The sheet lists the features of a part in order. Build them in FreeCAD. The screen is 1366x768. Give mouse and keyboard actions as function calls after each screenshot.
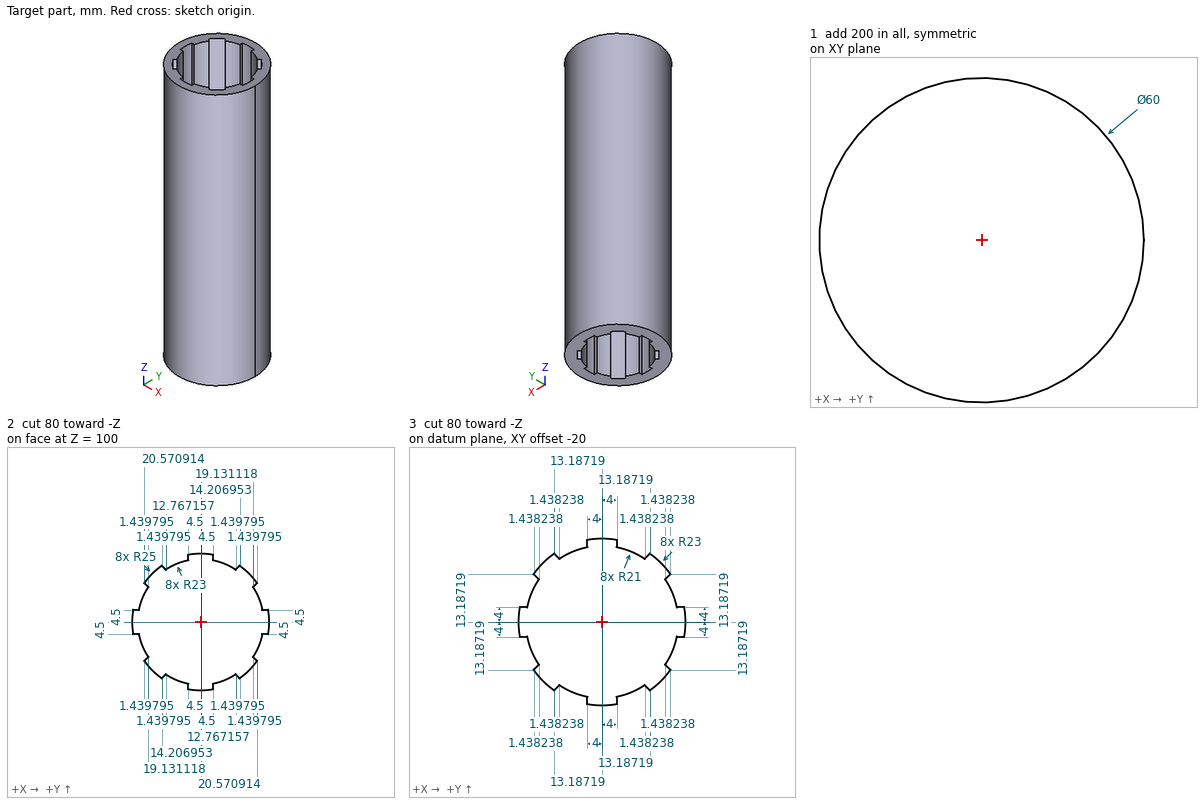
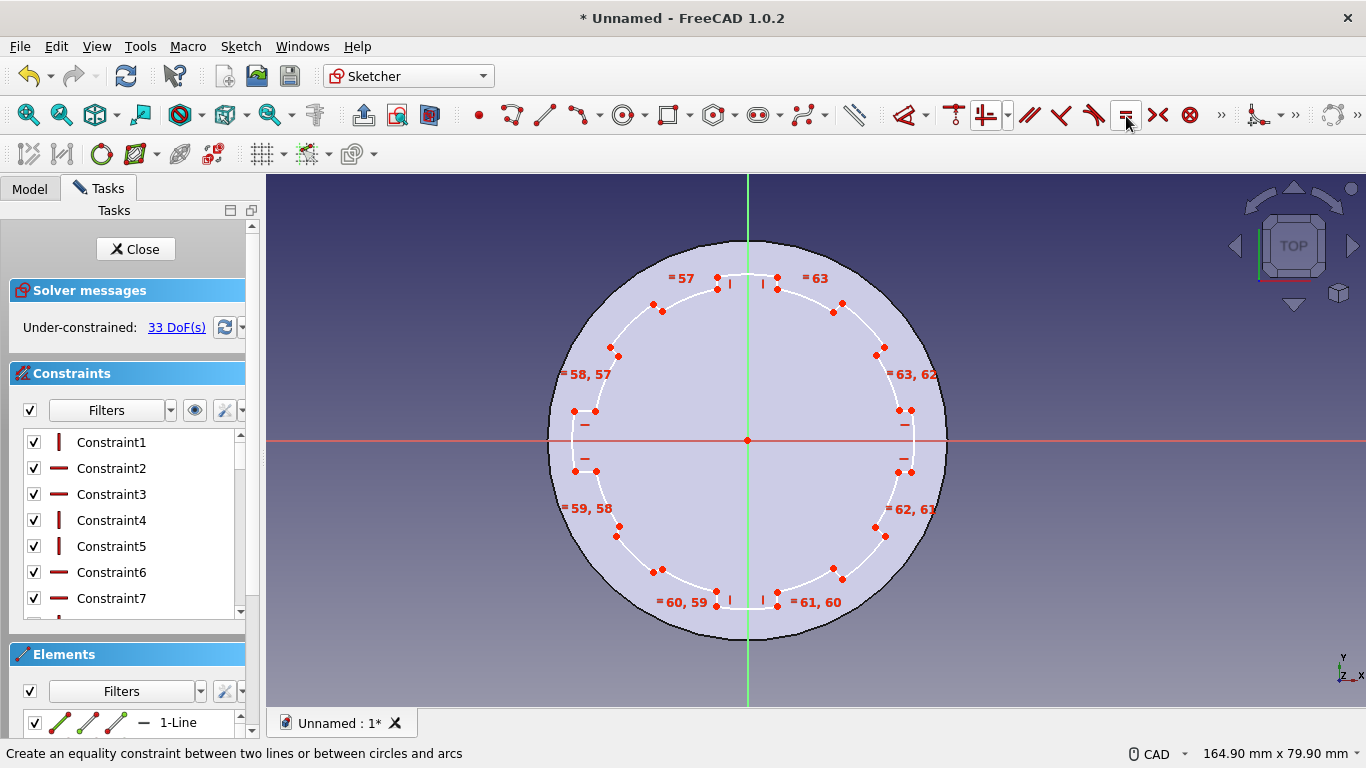
click(639, 315)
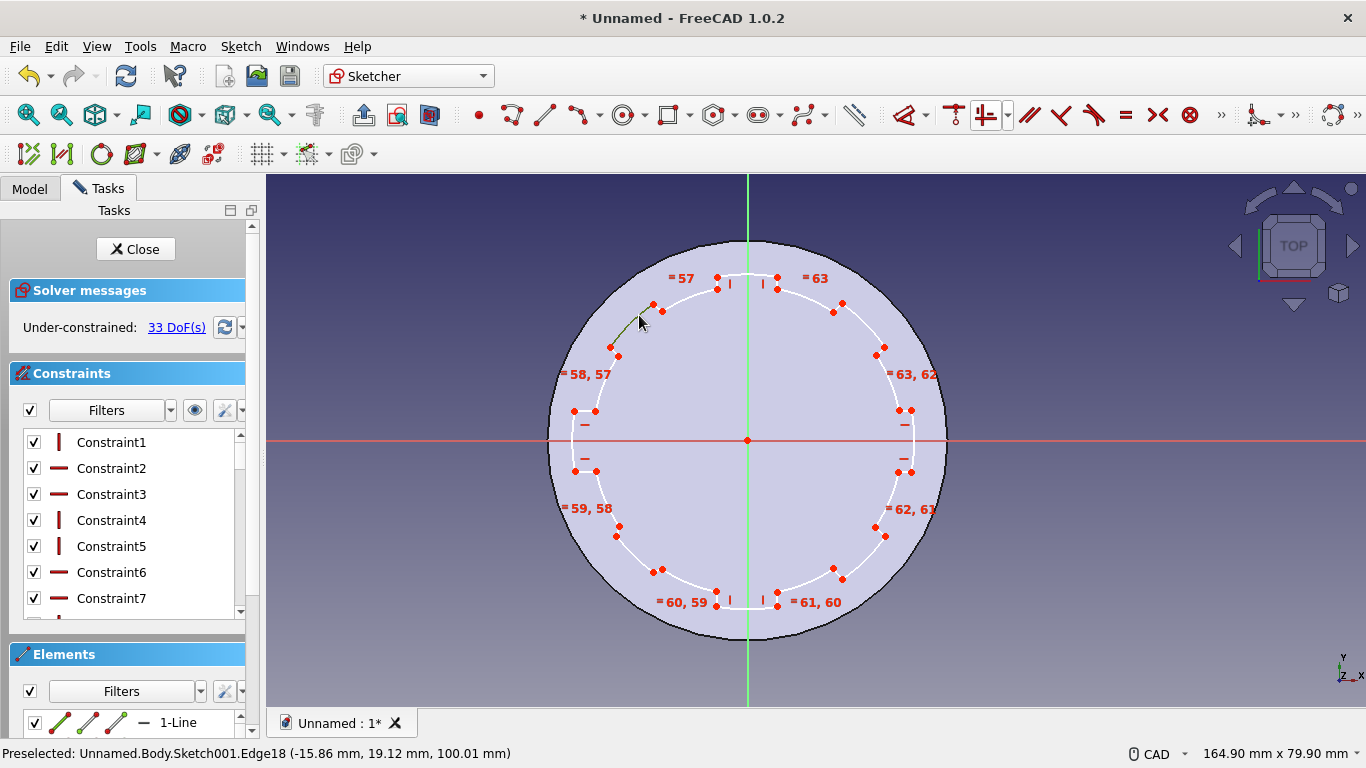
scroll(573, 429, up, 2)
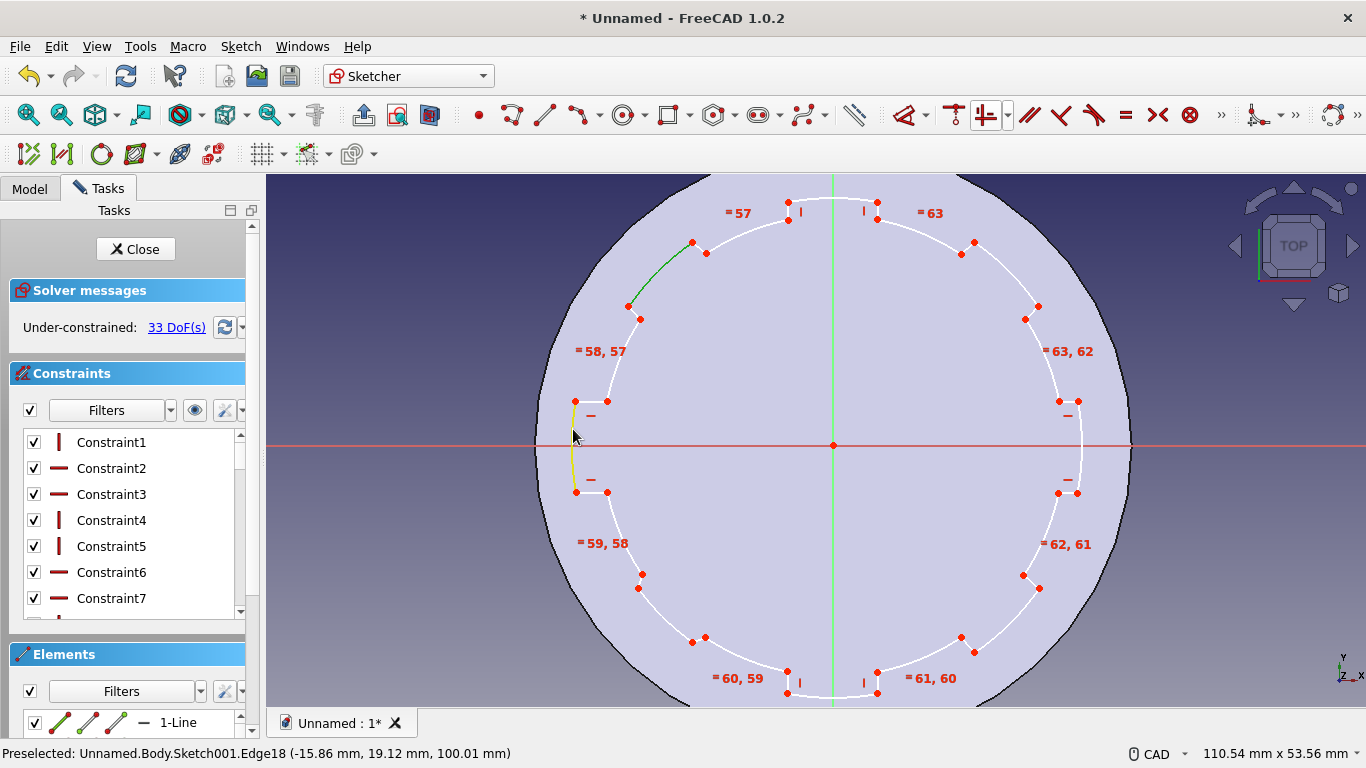
click(572, 429)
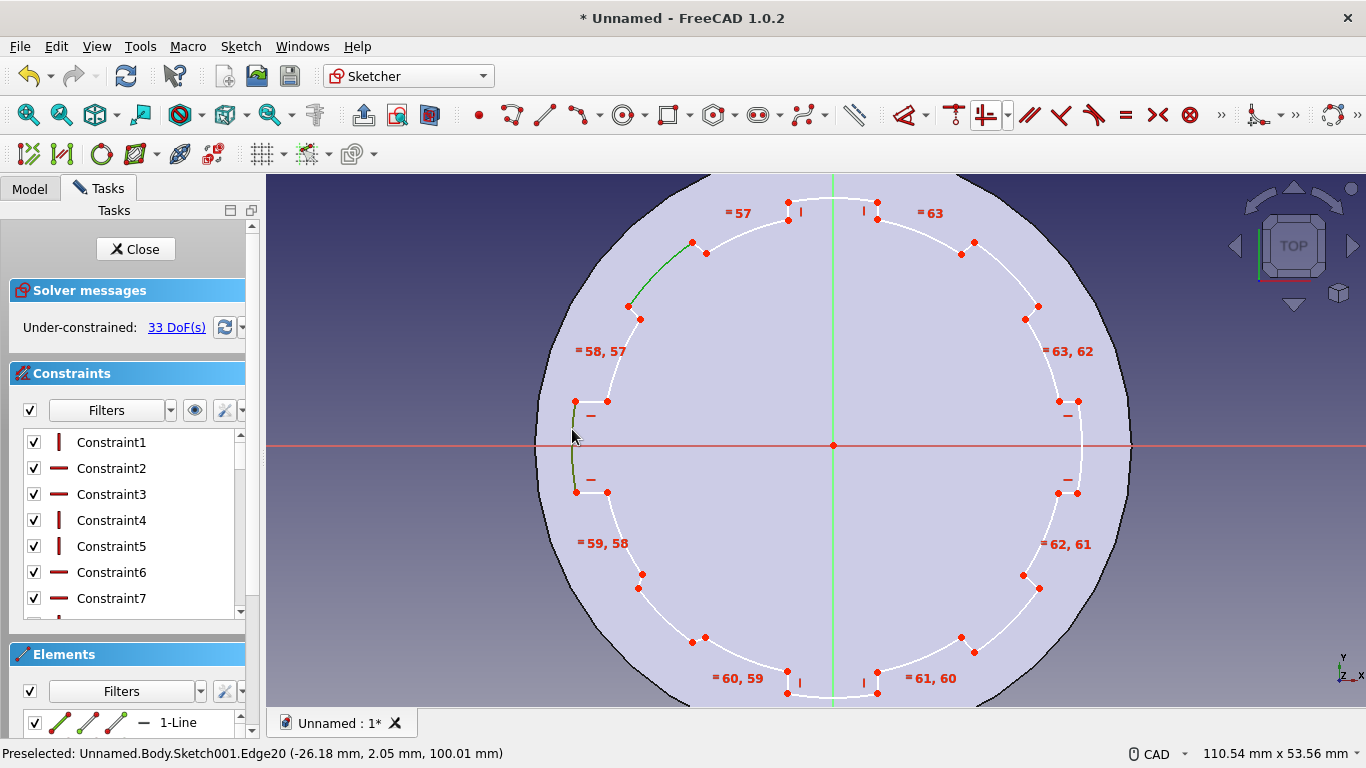
click(653, 606)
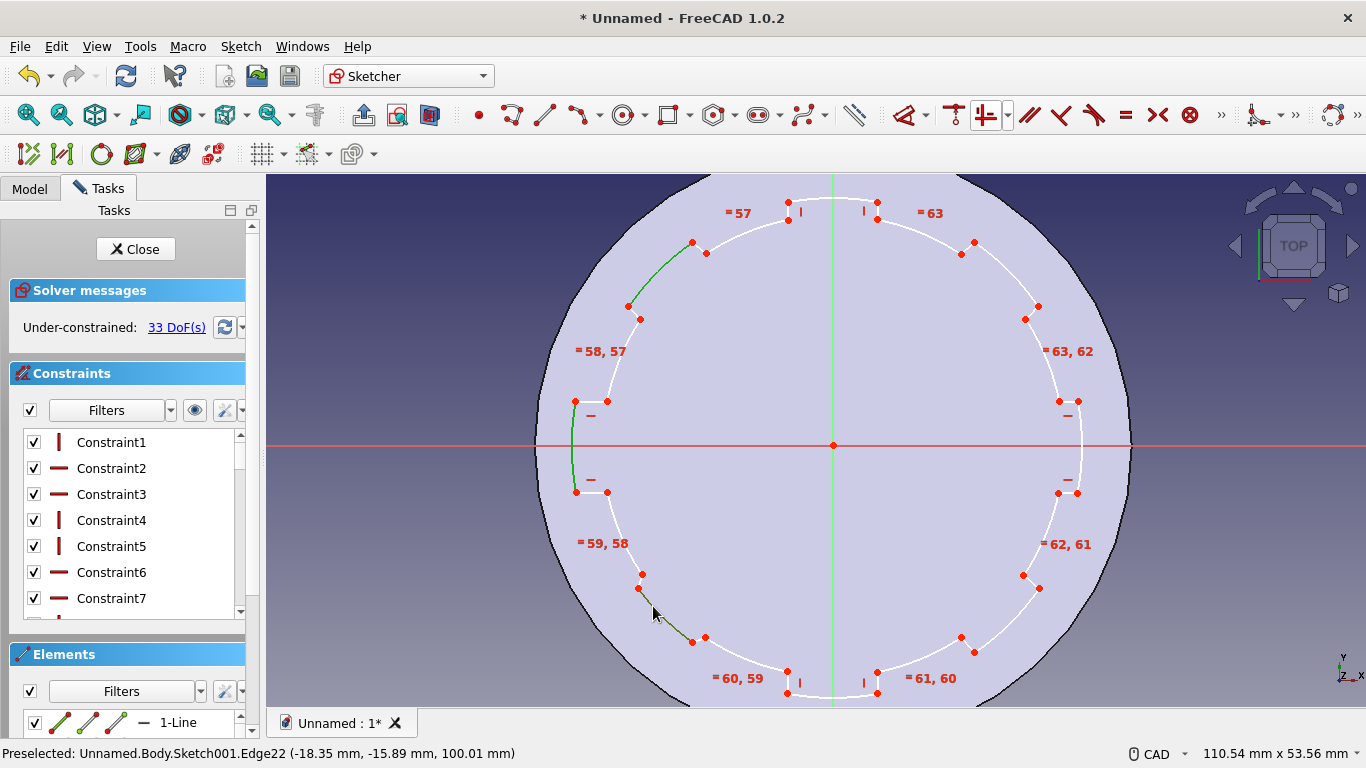
scroll(573, 429, down, 2)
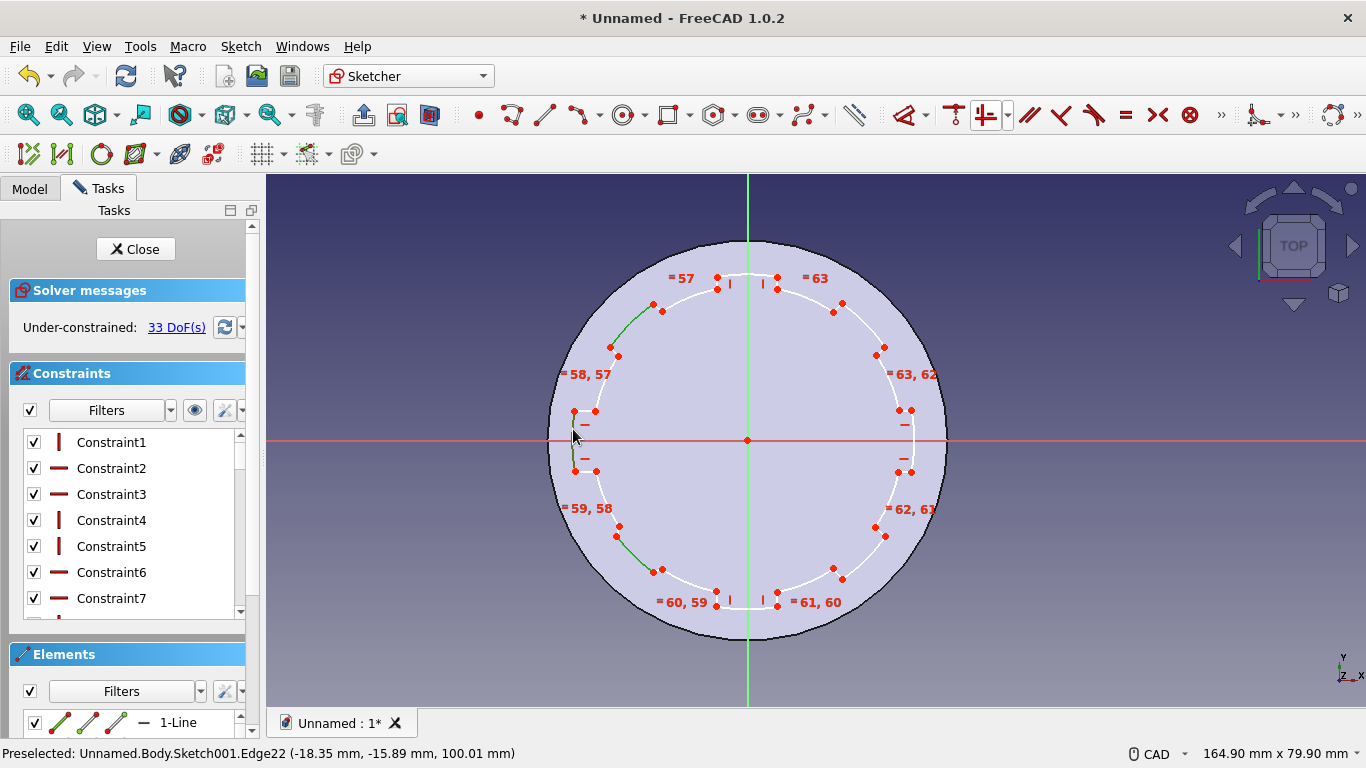
click(735, 609)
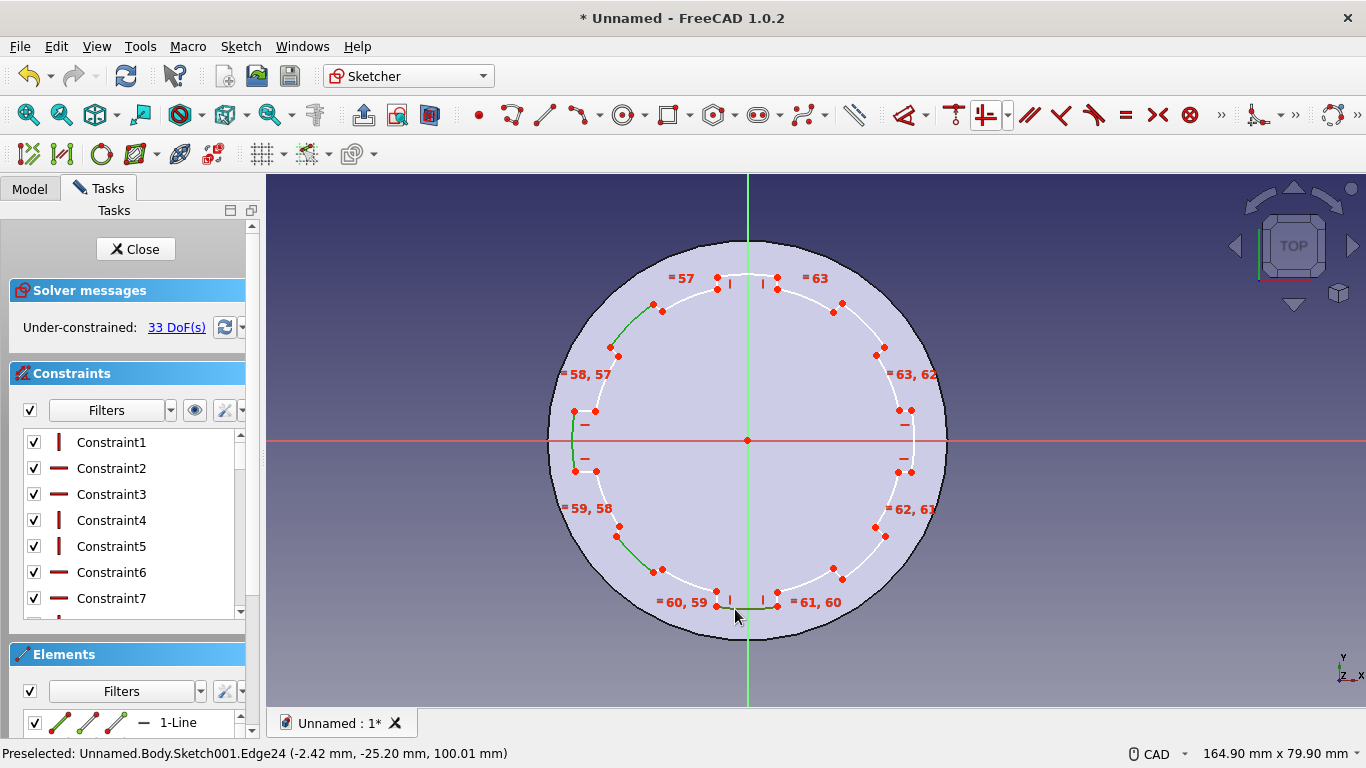
click(857, 568)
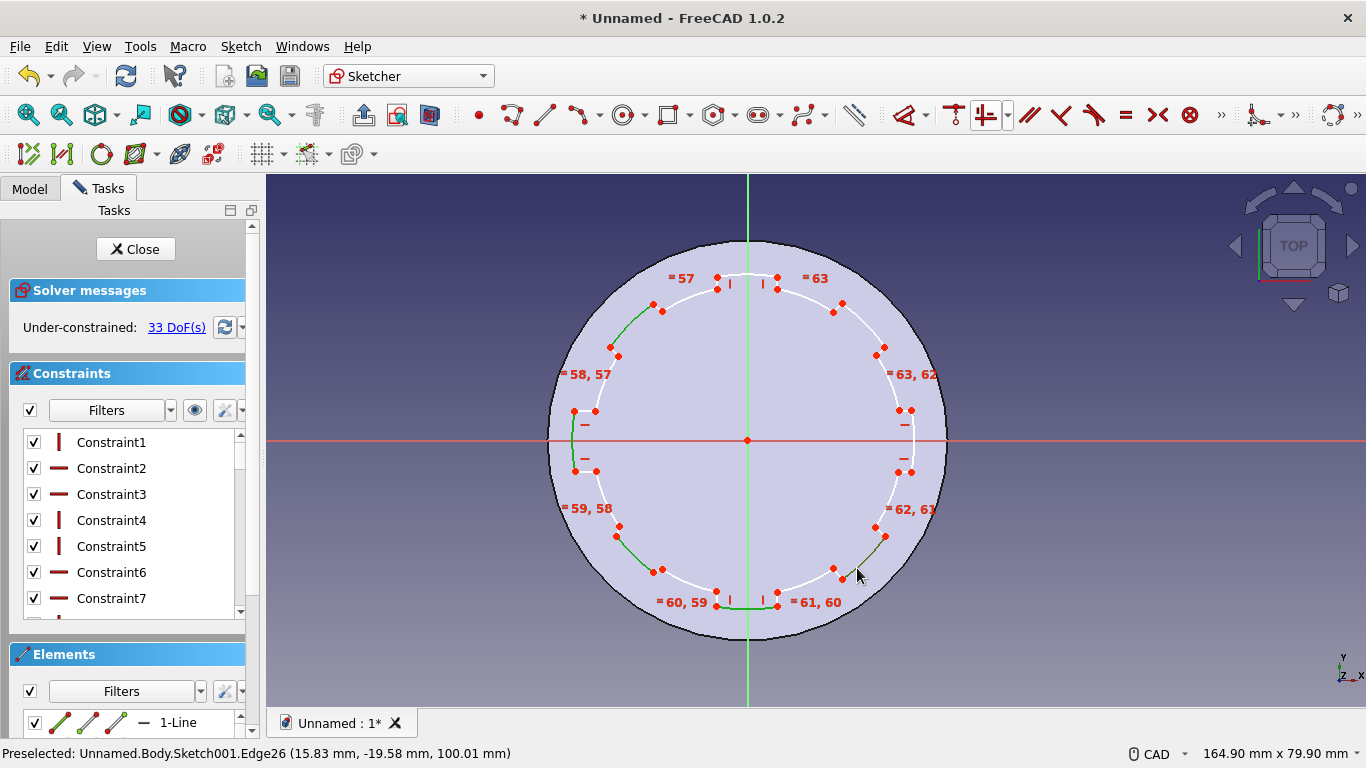
click(914, 454)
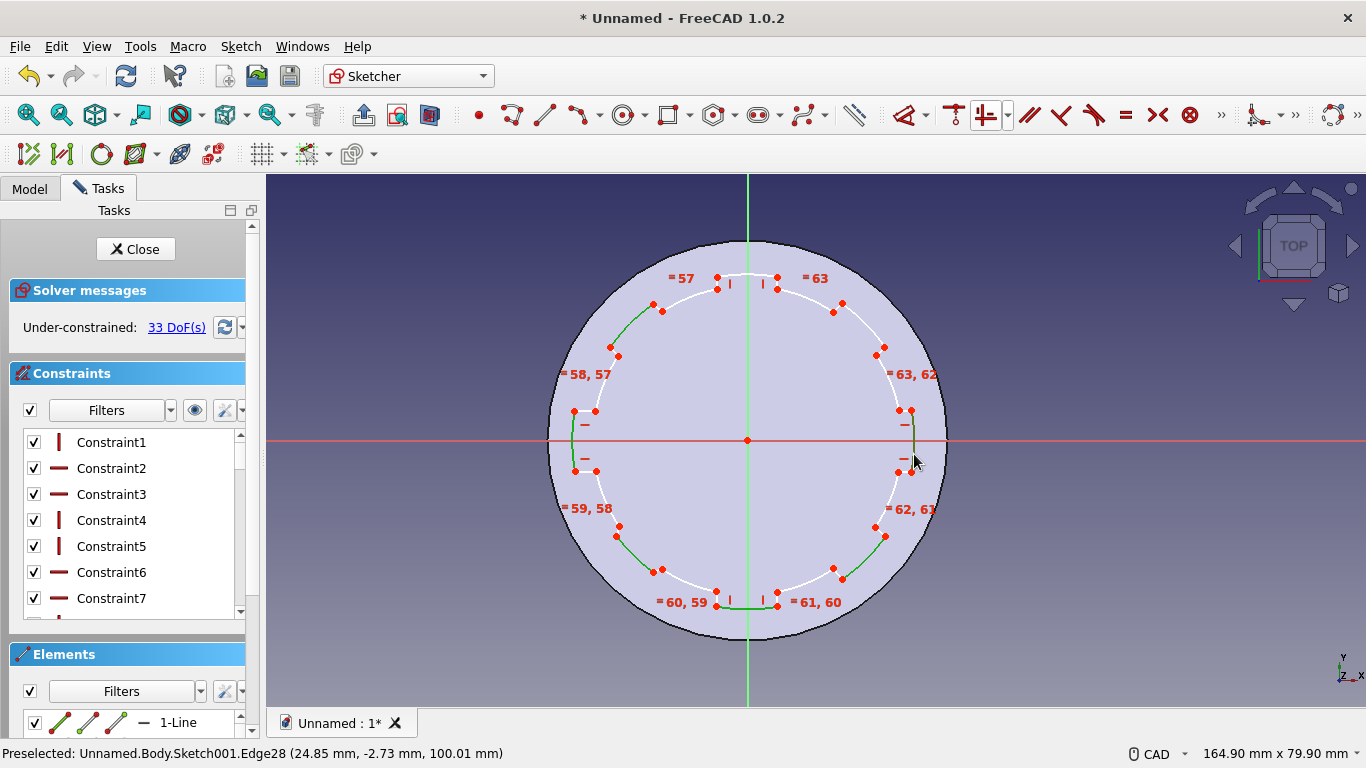
click(874, 333)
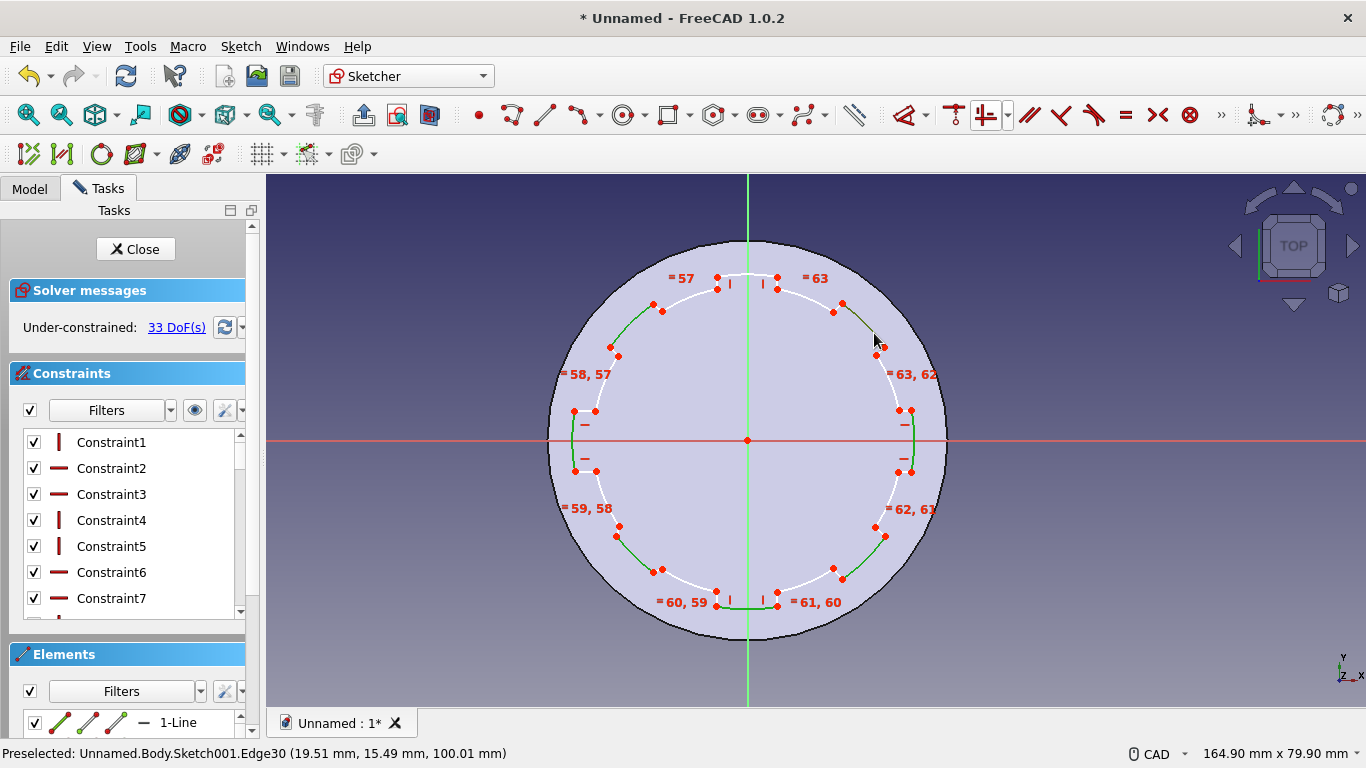
click(759, 275)